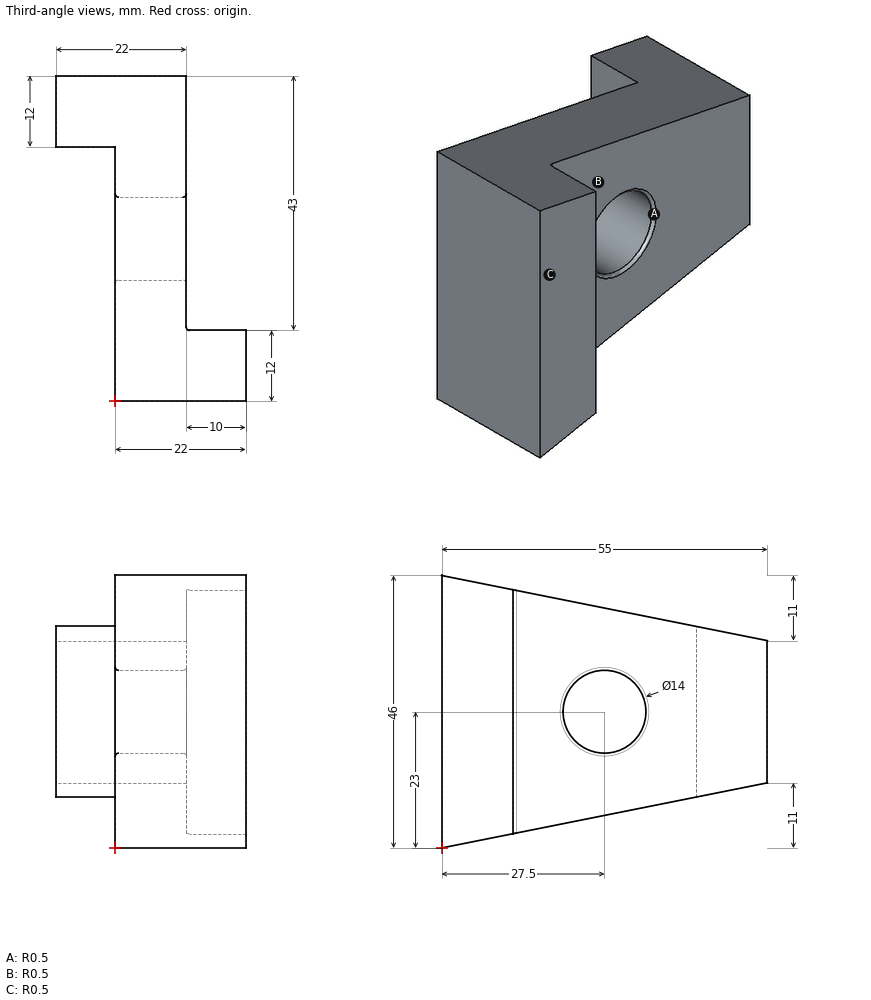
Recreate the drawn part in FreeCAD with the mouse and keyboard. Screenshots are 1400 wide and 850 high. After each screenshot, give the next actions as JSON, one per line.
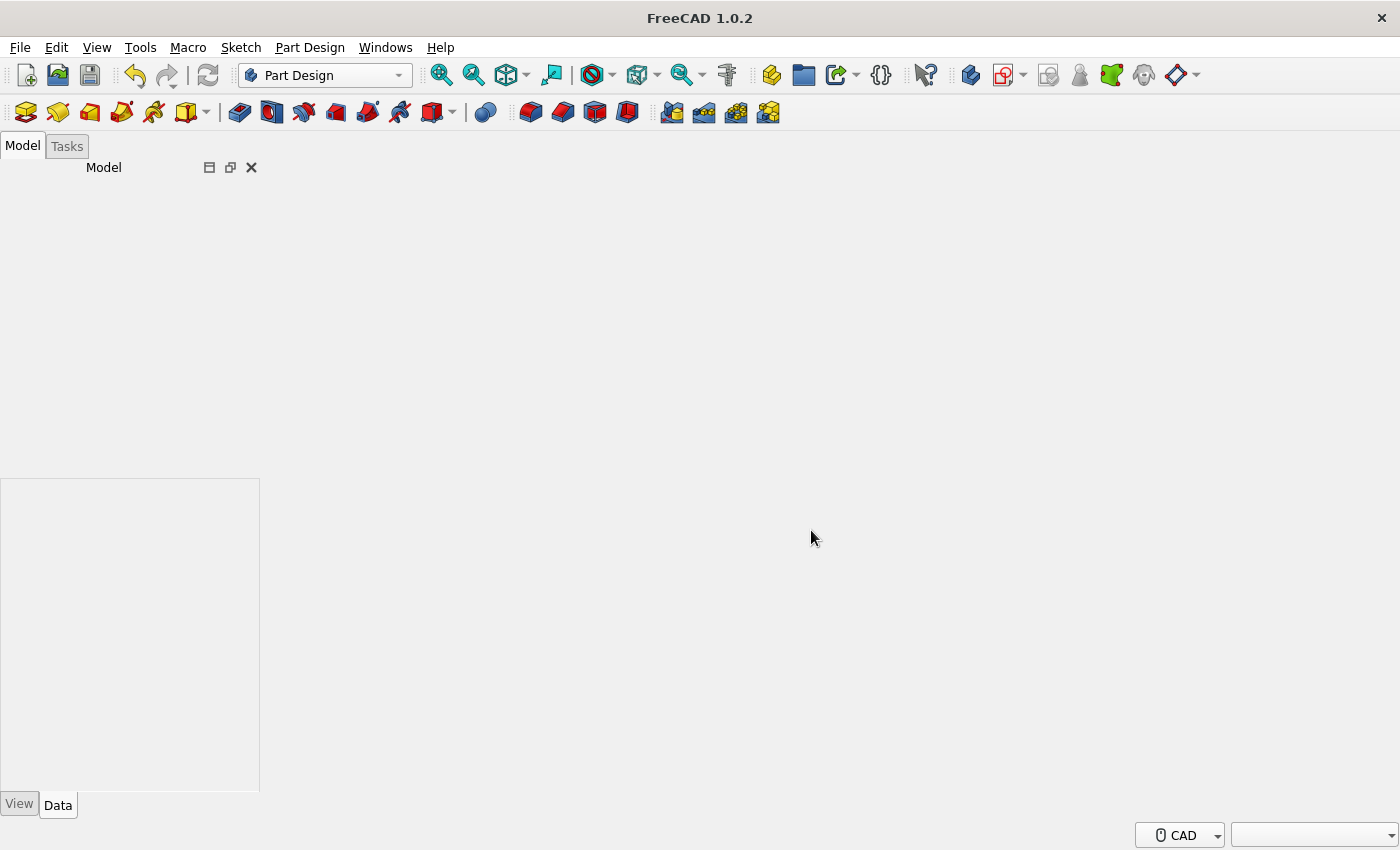
{"action": "left_click", "coordinate": [26, 76]}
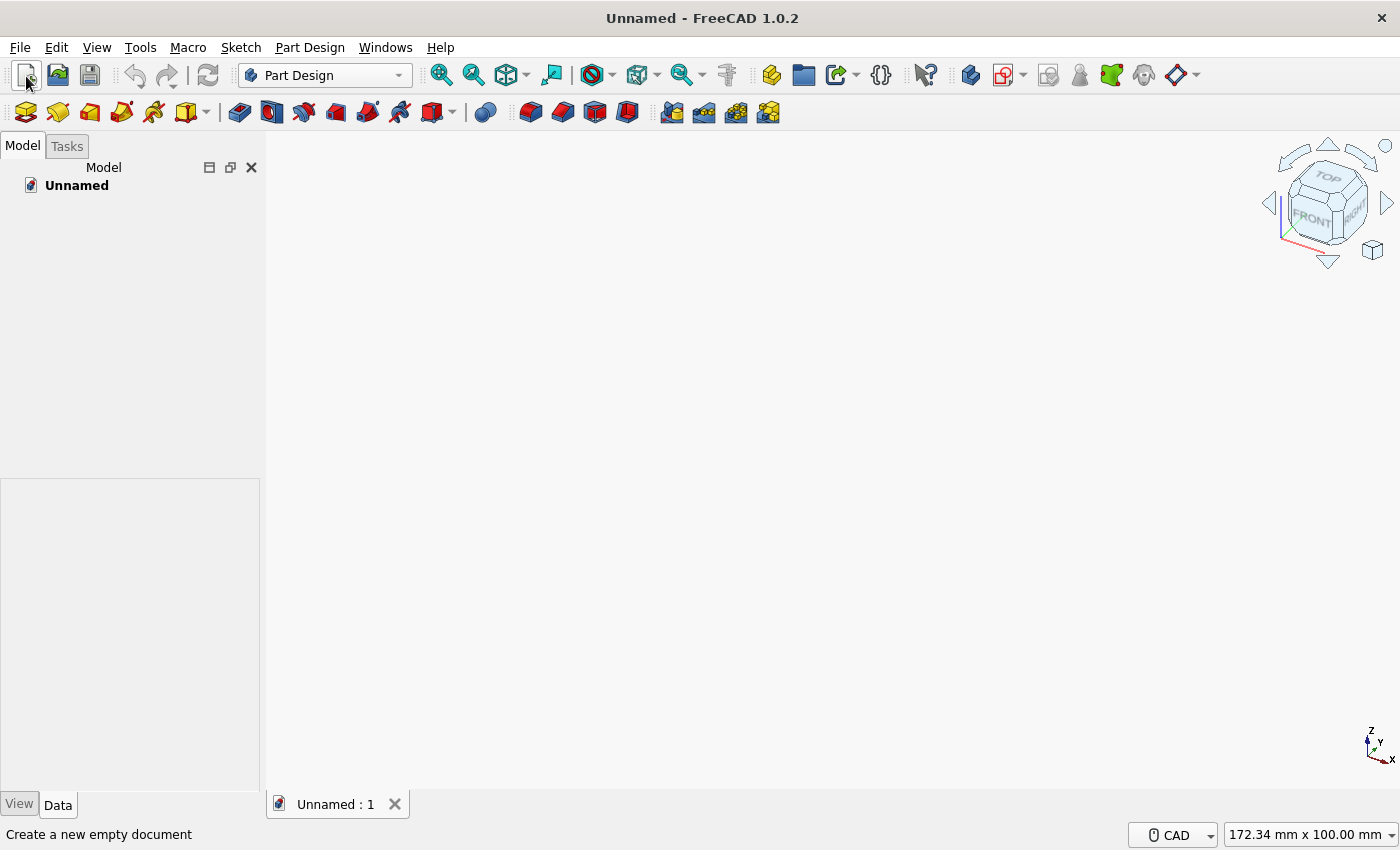
{"action": "left_click", "coordinate": [1004, 76]}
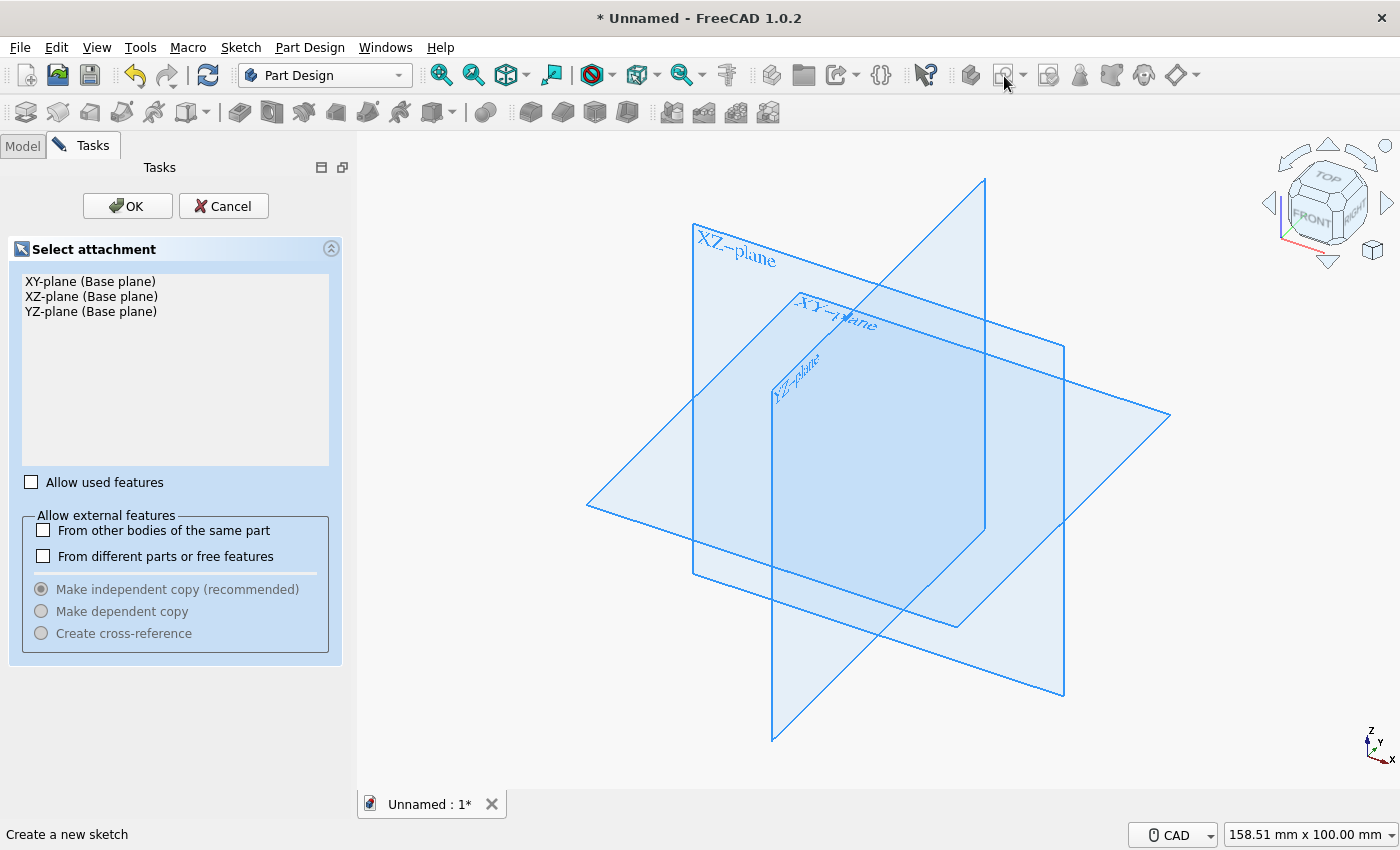
{"action": "left_click", "coordinate": [82, 282]}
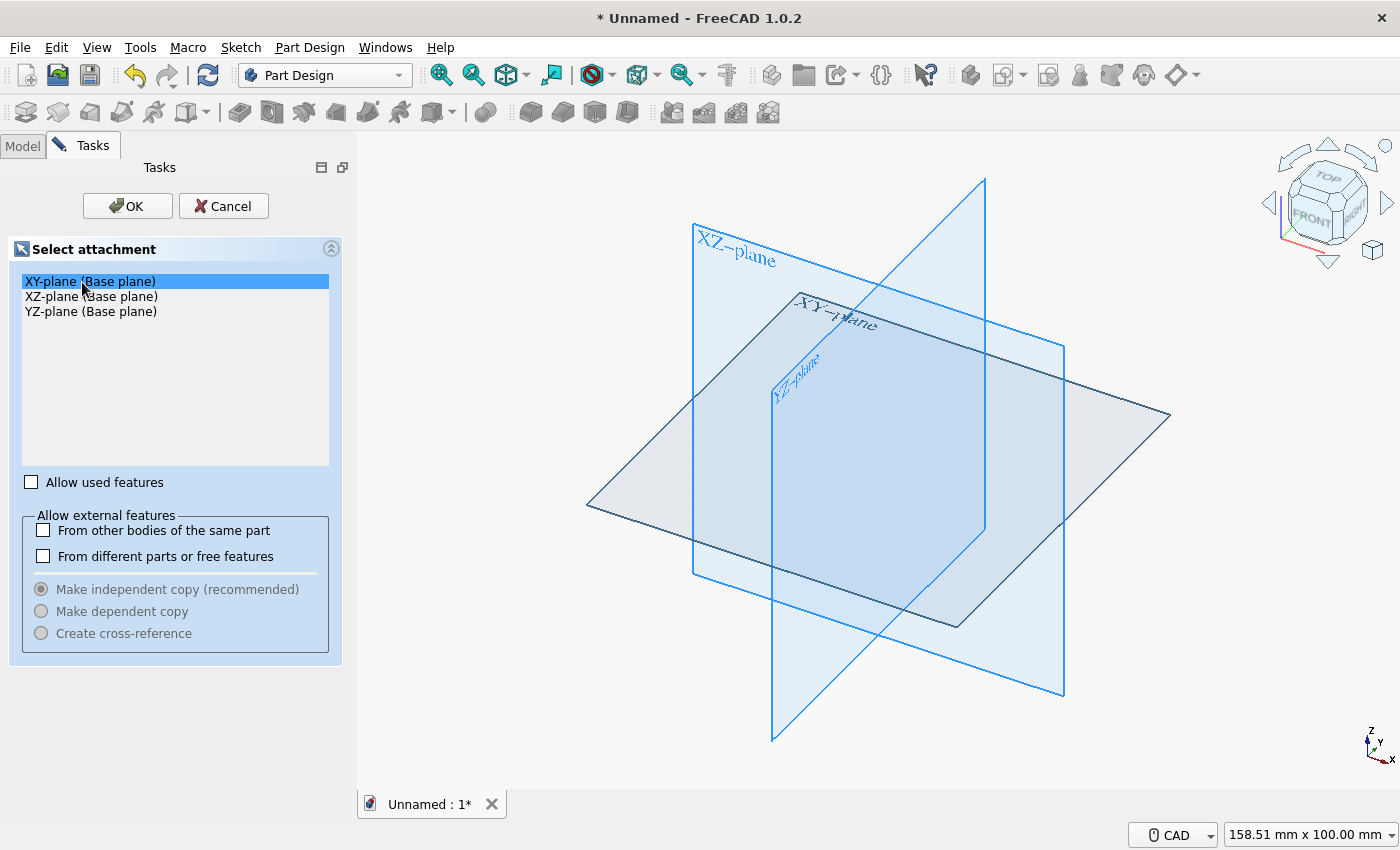
{"action": "left_click", "coordinate": [128, 206]}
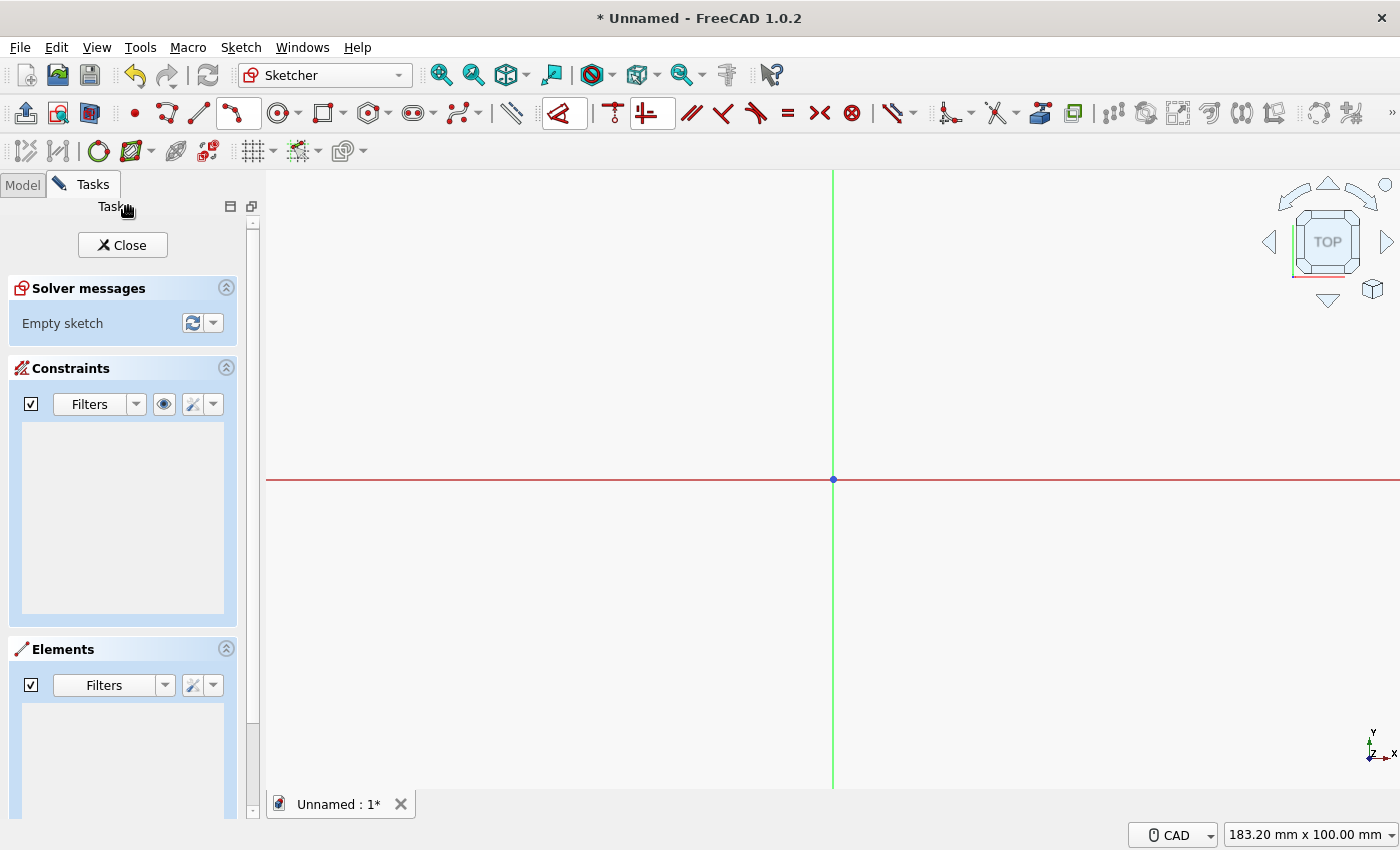
{"action": "scroll", "coordinate": [294, 761], "scroll_direction": "down", "scroll_amount": 1}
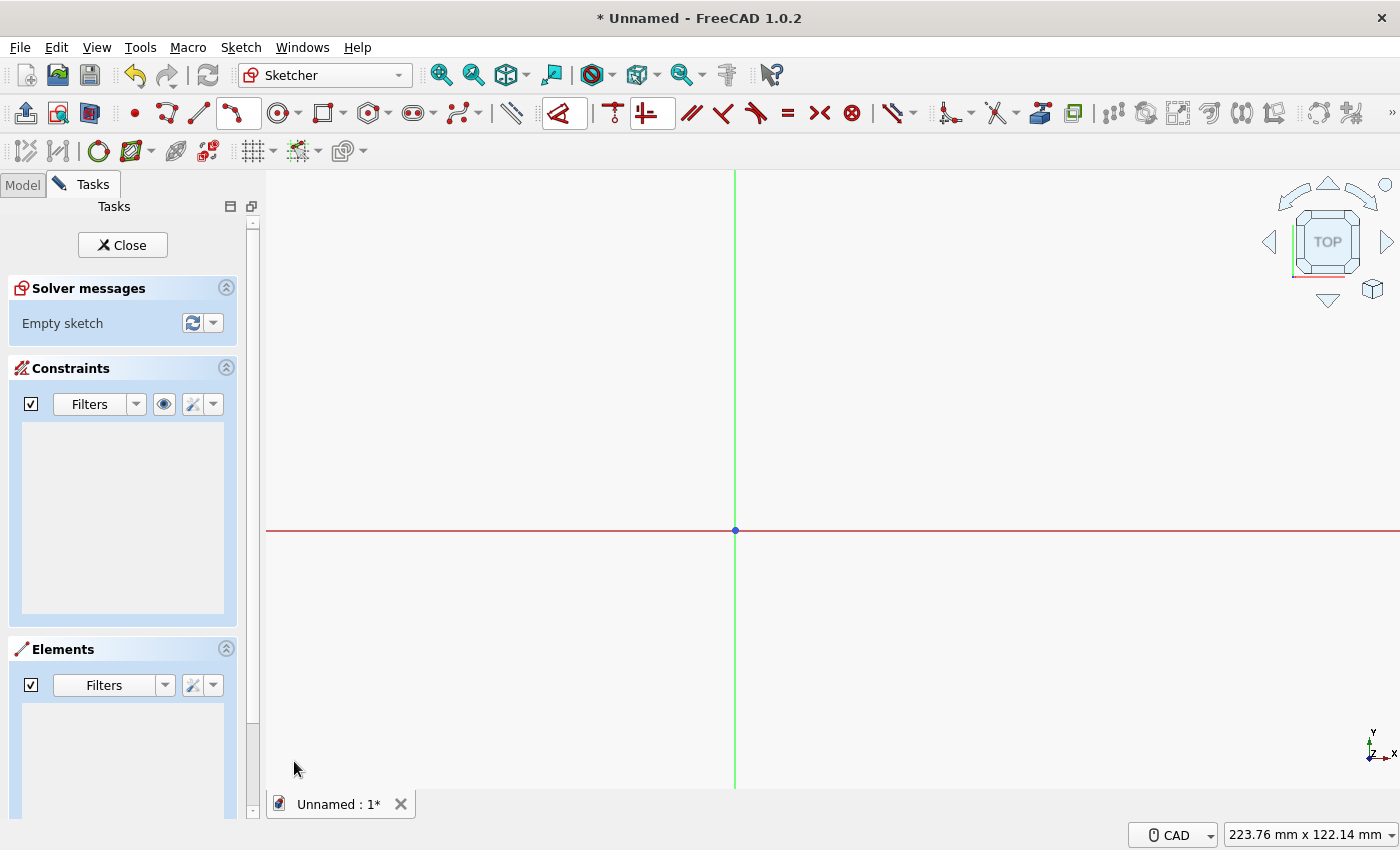
{"action": "scroll", "coordinate": [768, 212], "scroll_direction": "up", "scroll_amount": 2}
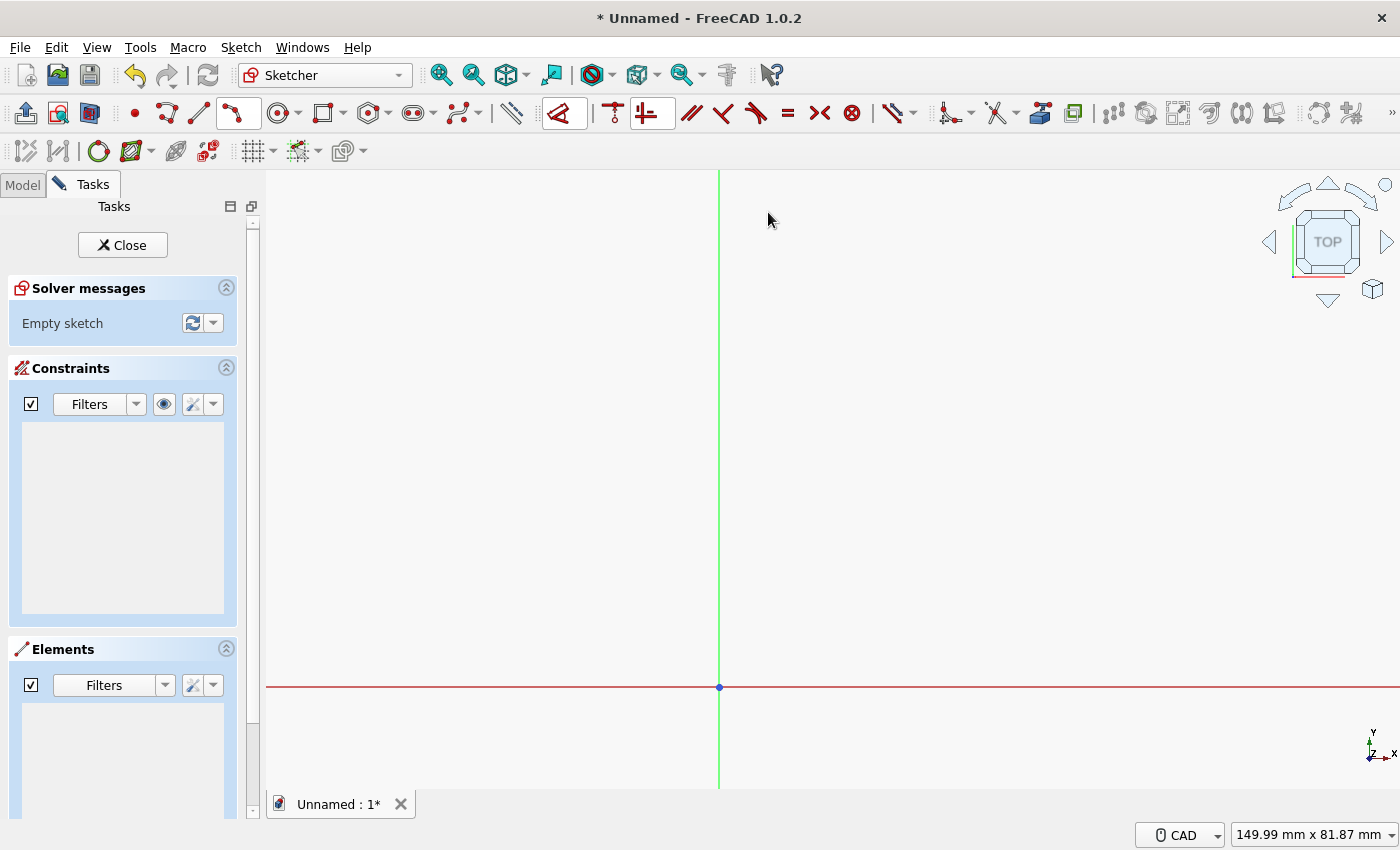
{"action": "left_click", "coordinate": [168, 114]}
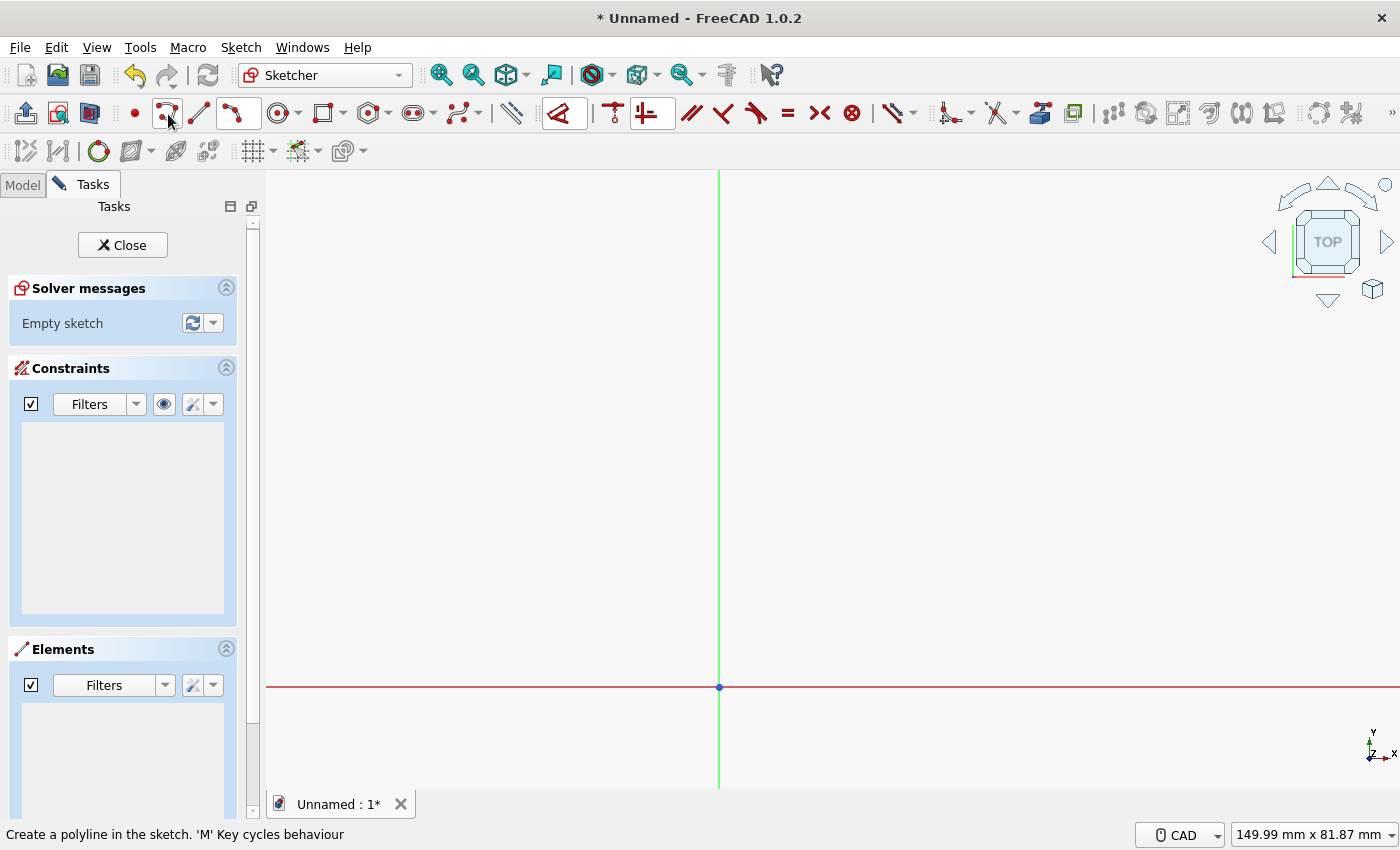
{"action": "left_click", "coordinate": [719, 687]}
{"action": "left_click", "coordinate": [885, 678]}
{"action": "left_click", "coordinate": [885, 597]}
{"action": "left_click", "coordinate": [810, 597]}
{"action": "left_click", "coordinate": [810, 272]}
{"action": "left_click", "coordinate": [643, 272]}
{"action": "left_click", "coordinate": [643, 362]}
{"action": "left_click", "coordinate": [728, 362]}
{"action": "left_click", "coordinate": [719, 687]}
{"action": "key", "text": "Escape"}
{"action": "key", "text": "Escape"}